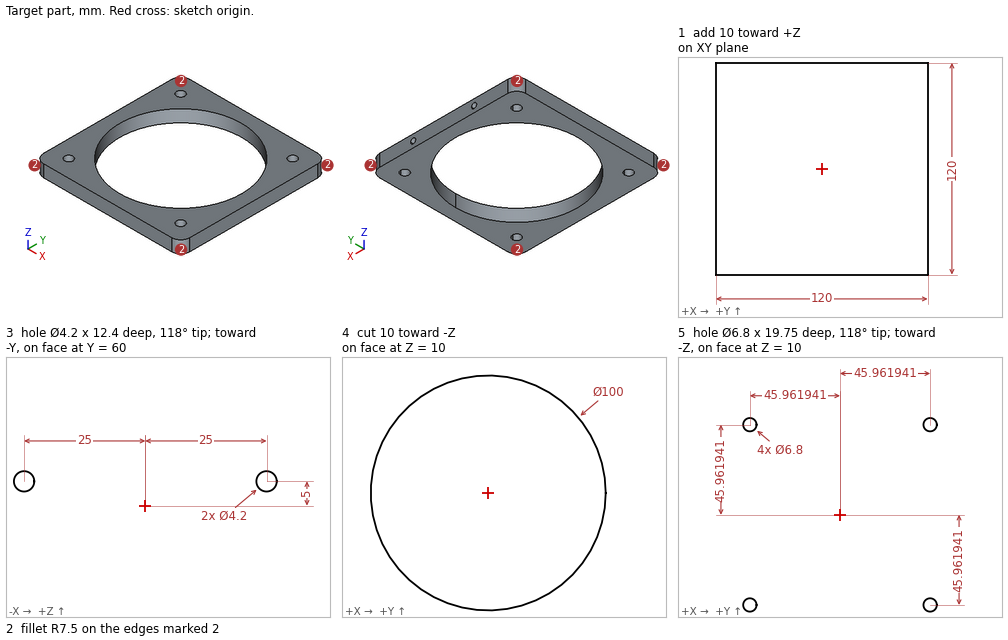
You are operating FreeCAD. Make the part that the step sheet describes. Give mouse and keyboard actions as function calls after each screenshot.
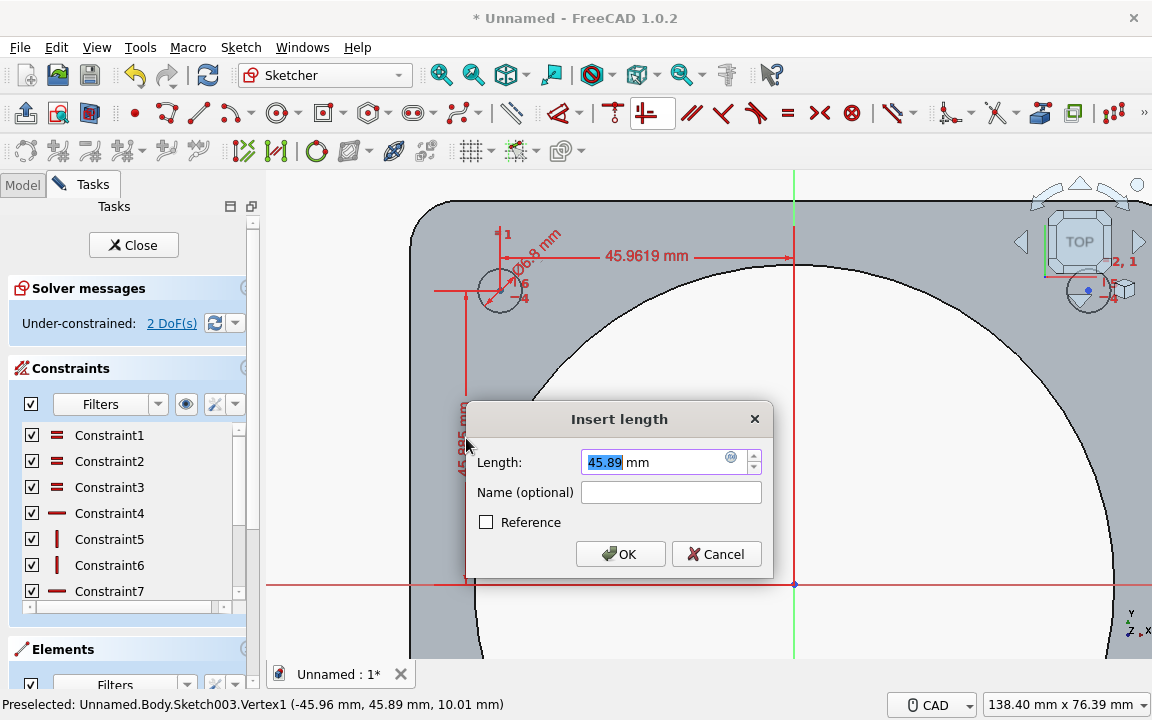
text(45.961941)
key(Return)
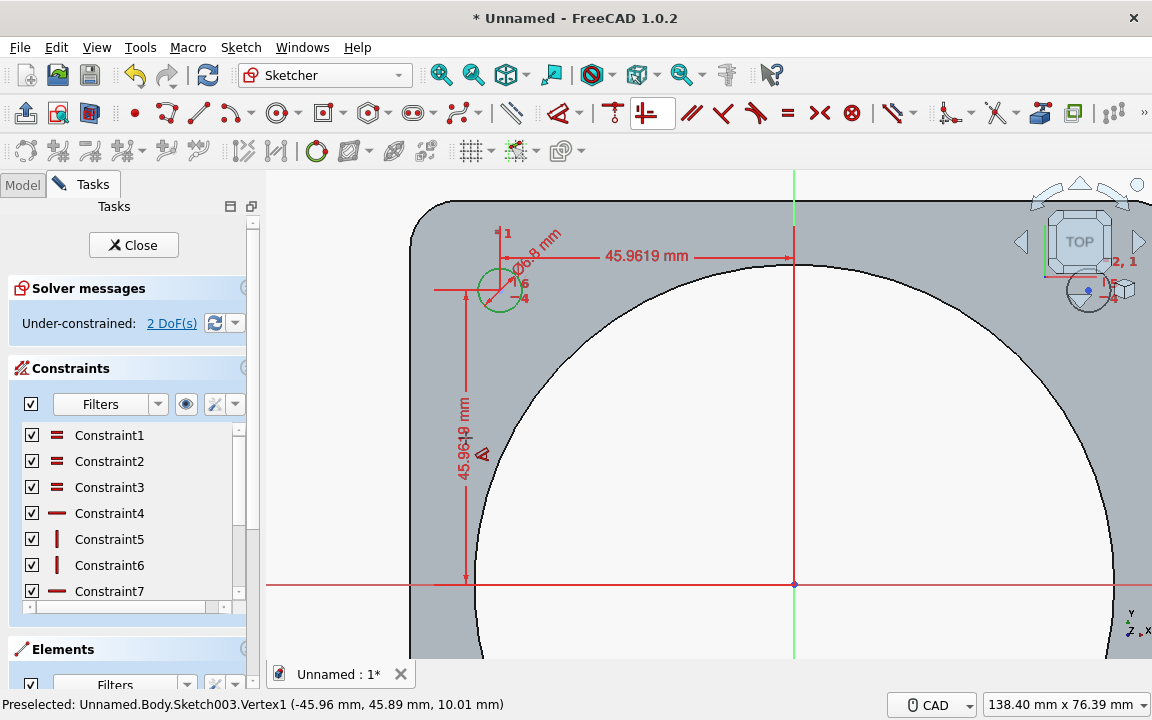
scroll(515, 276, down, 4)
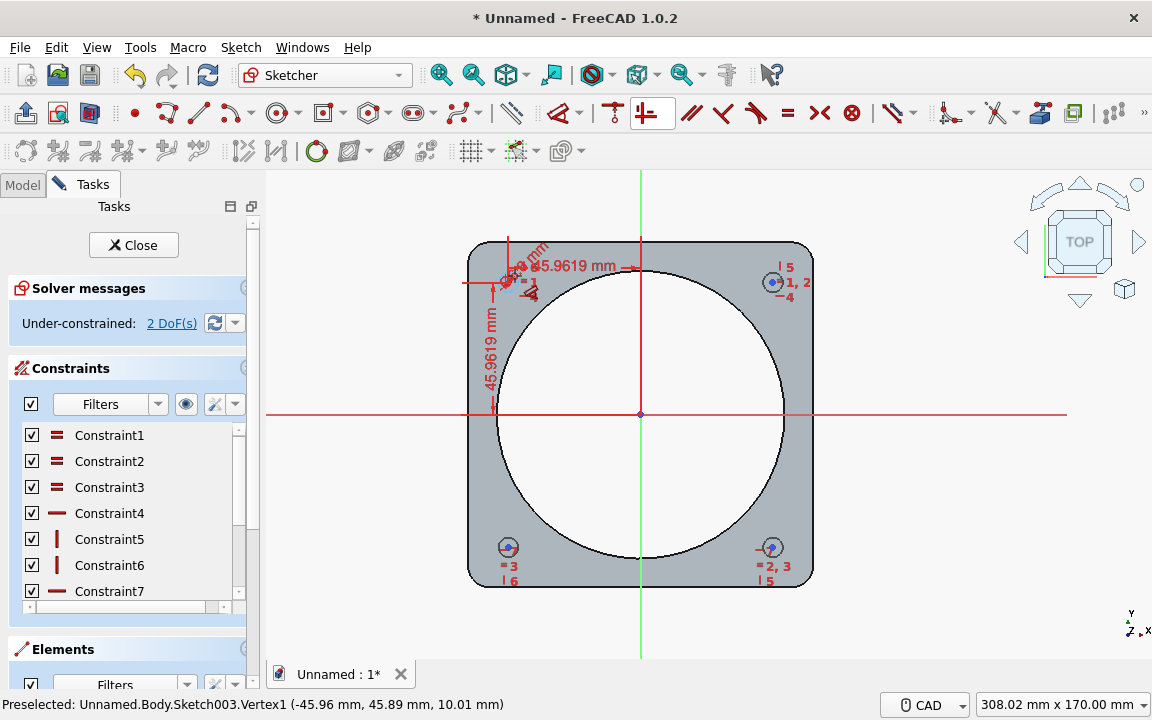
click(773, 283)
click(707, 249)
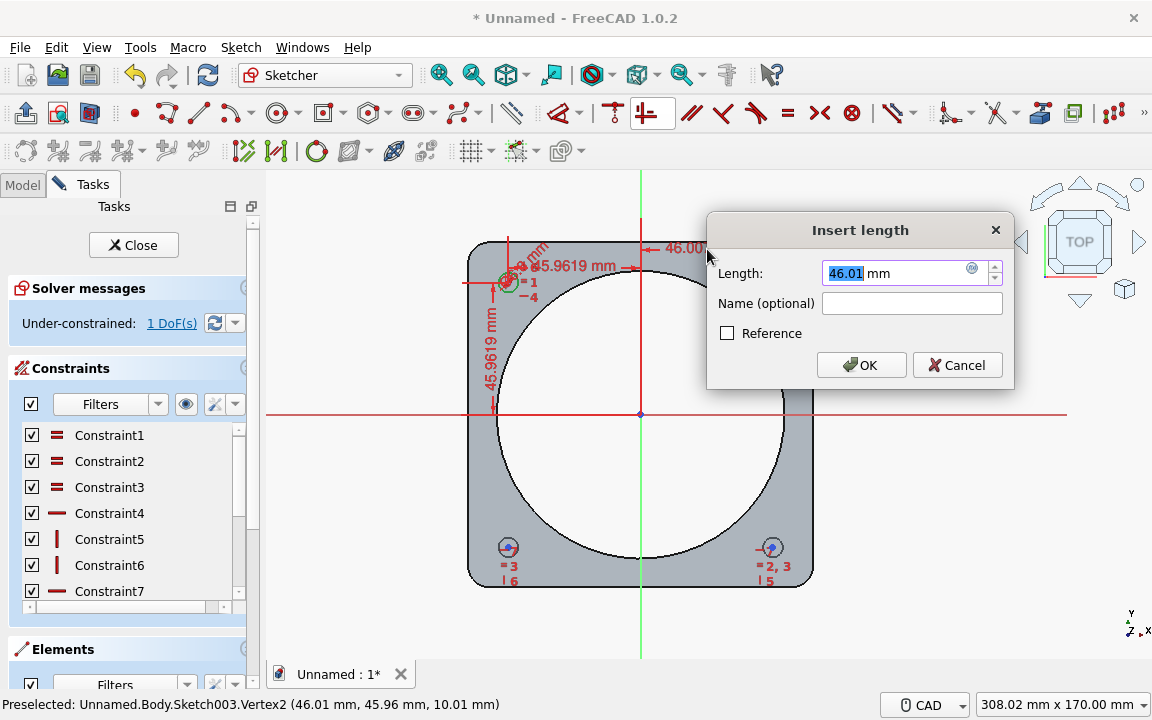
text(45.961941)
key(Return)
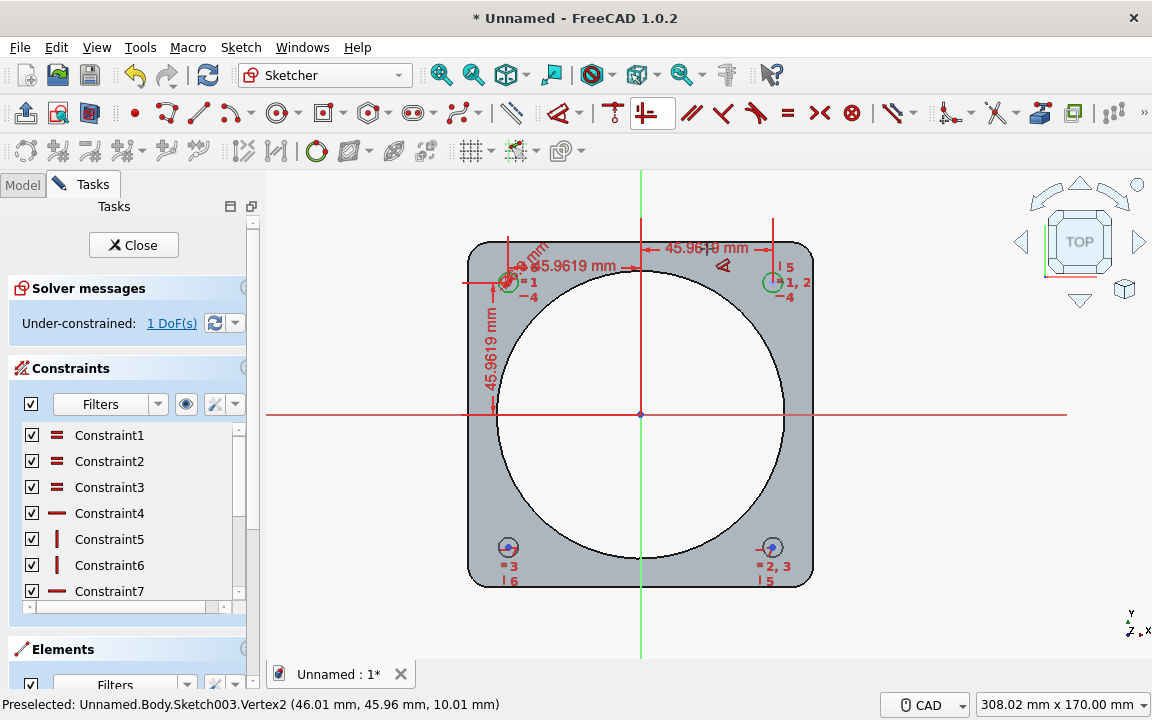
click(773, 547)
click(807, 481)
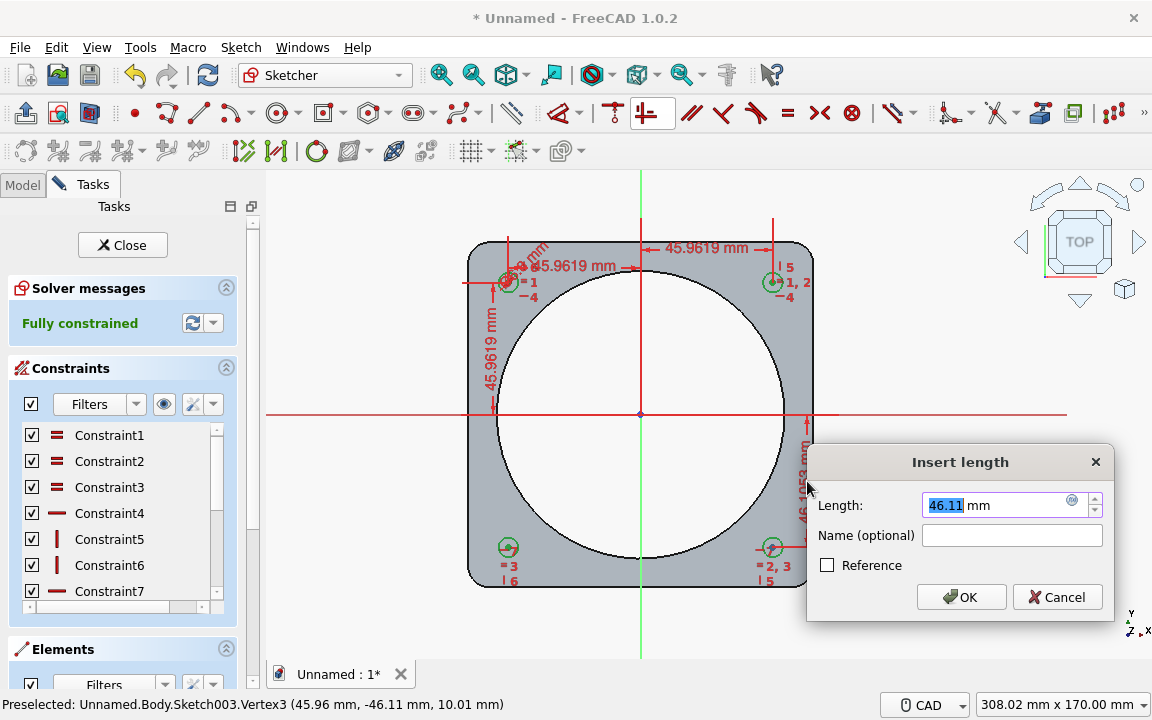
text(45.961941)
key(Return)
key(Escape)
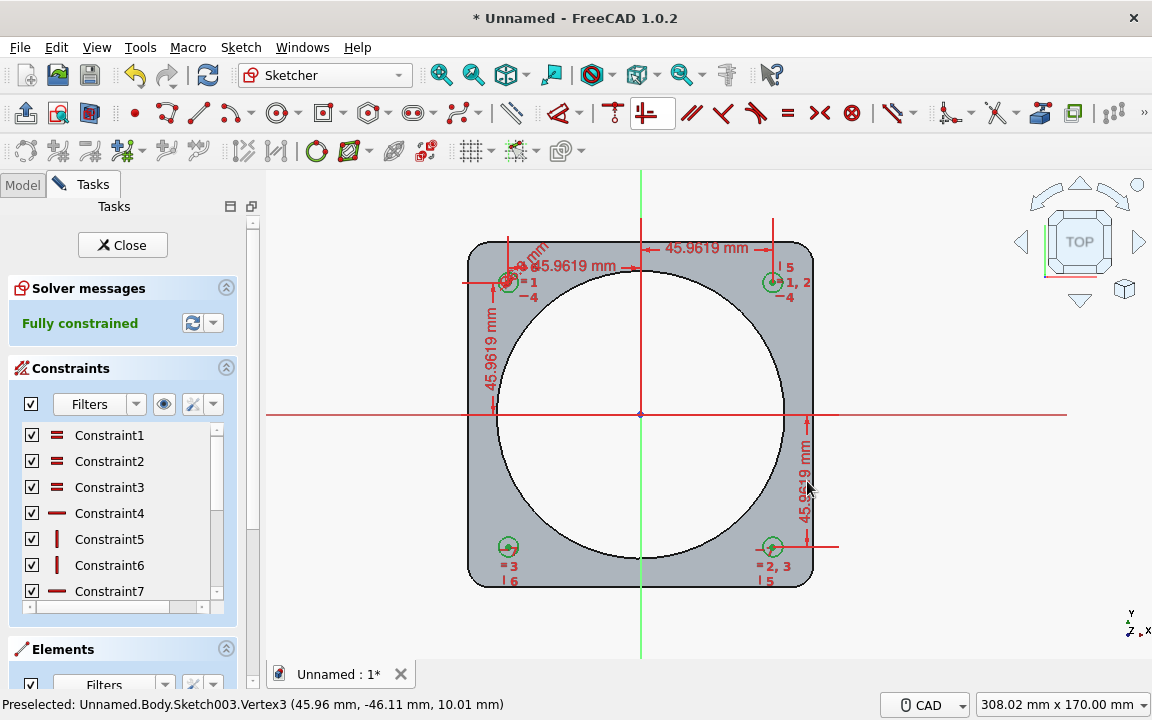
click(123, 245)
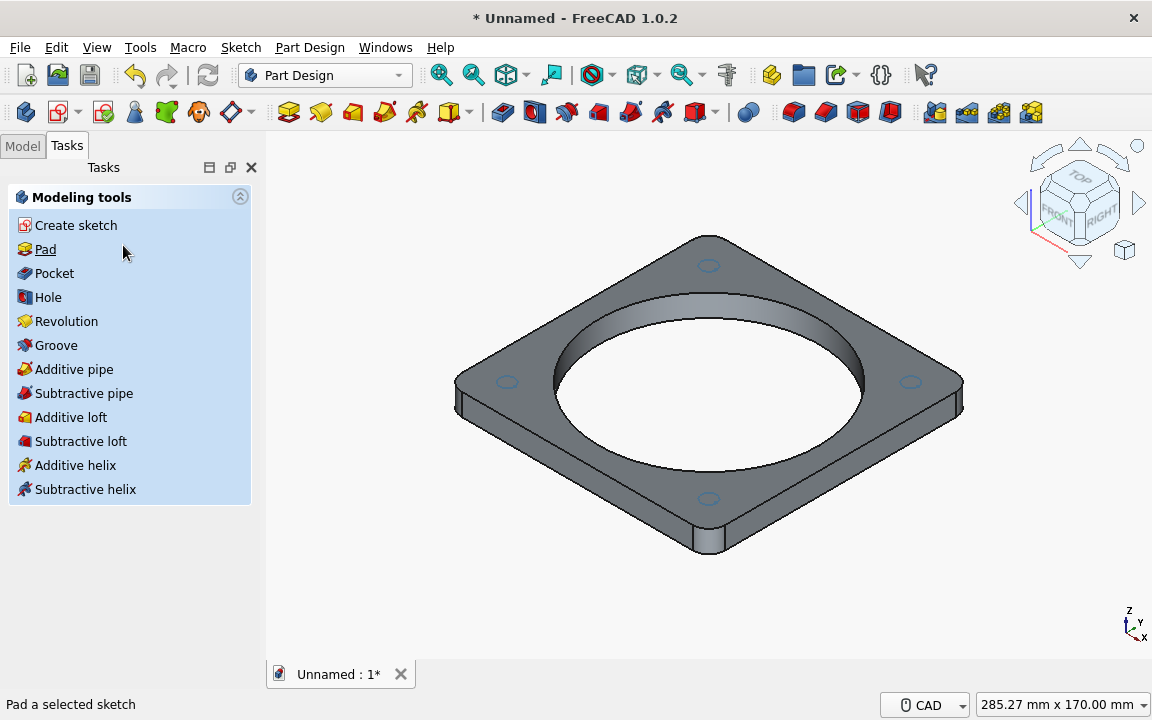
click(536, 112)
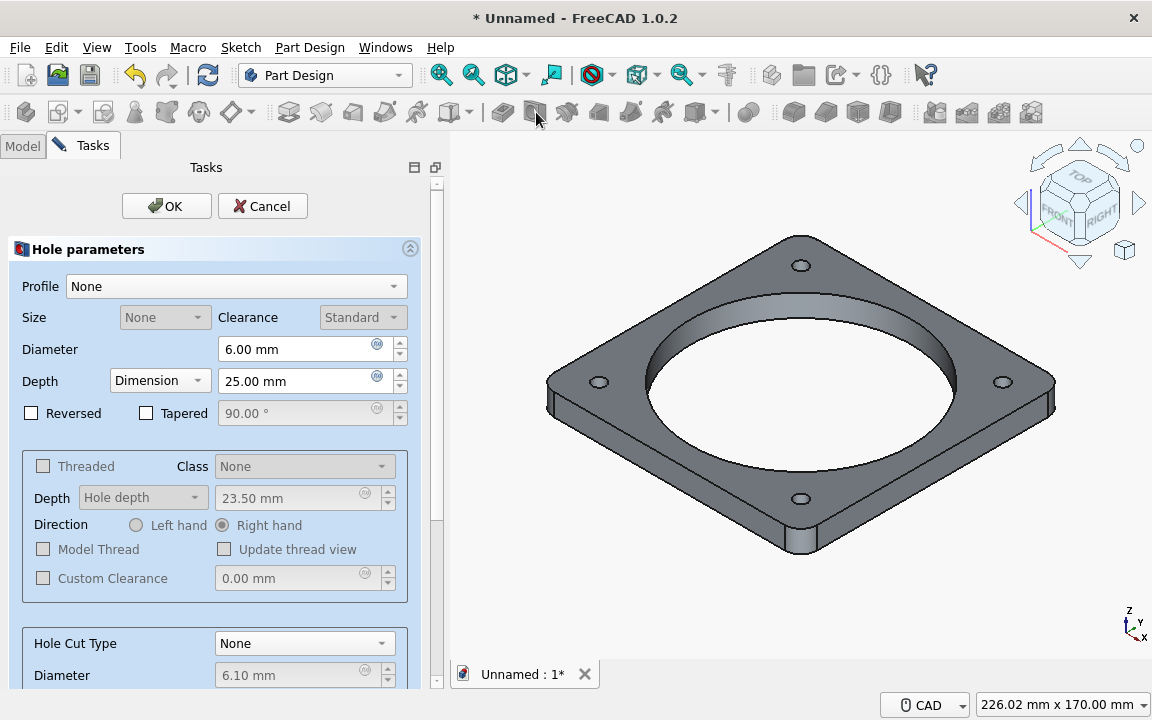
triple_click(305, 349)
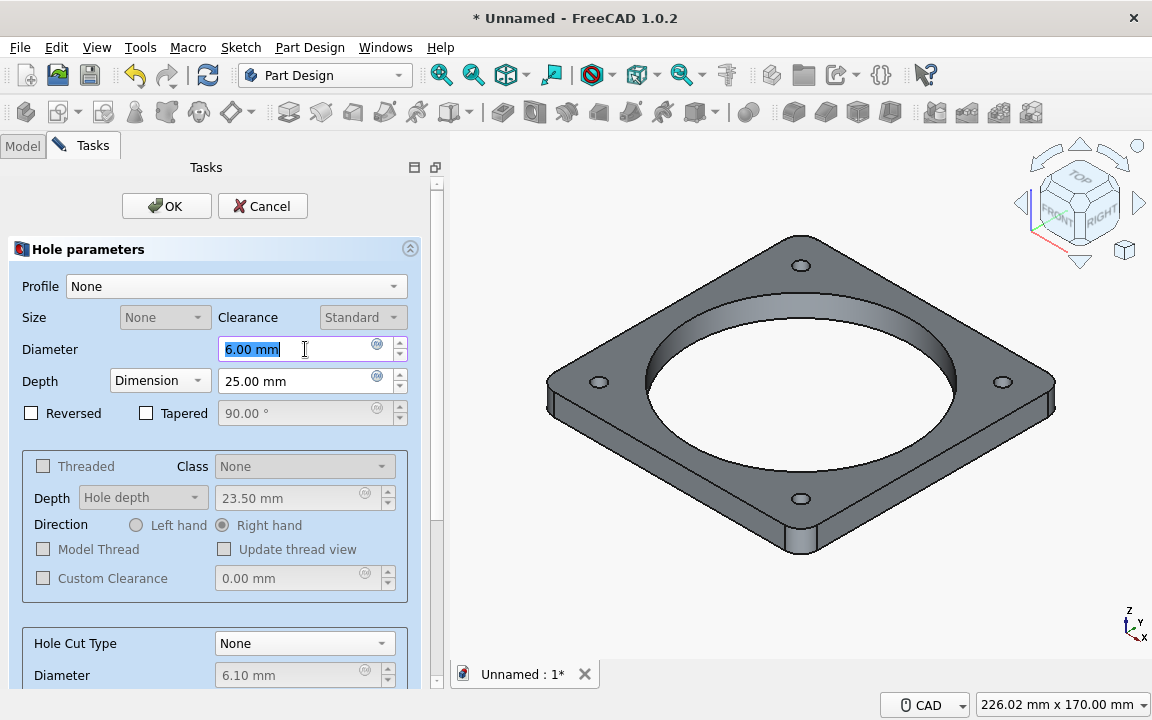
text(6.8)
key(Tab)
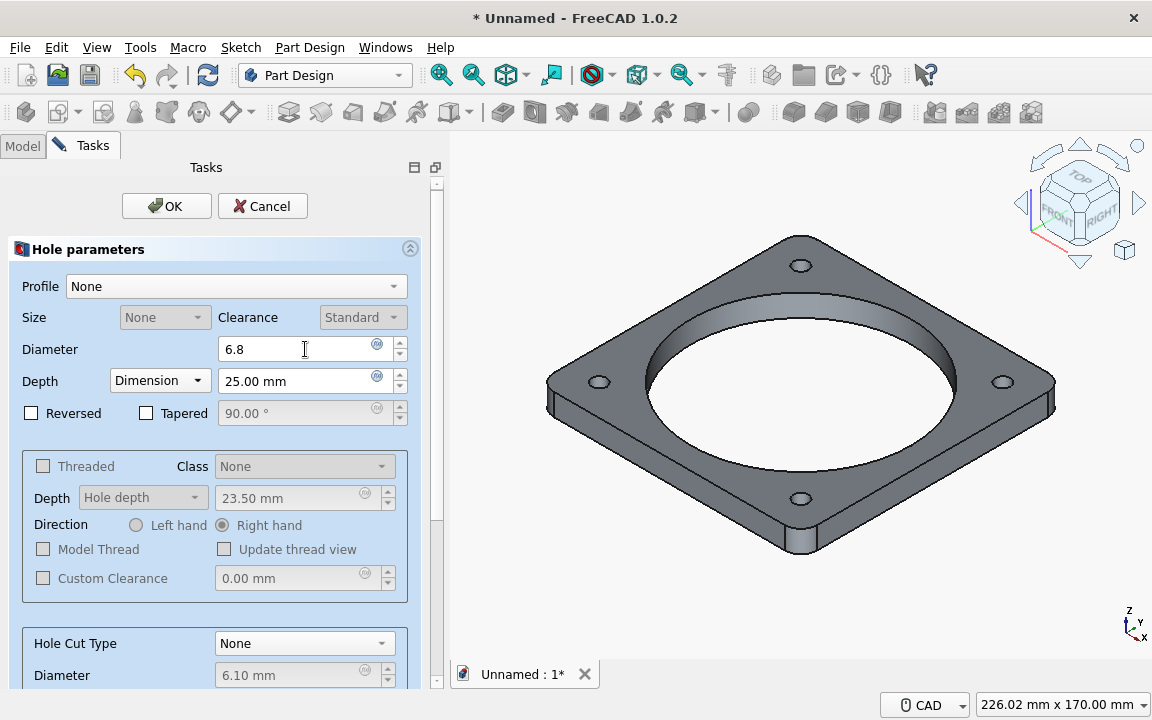
triple_click(305, 381)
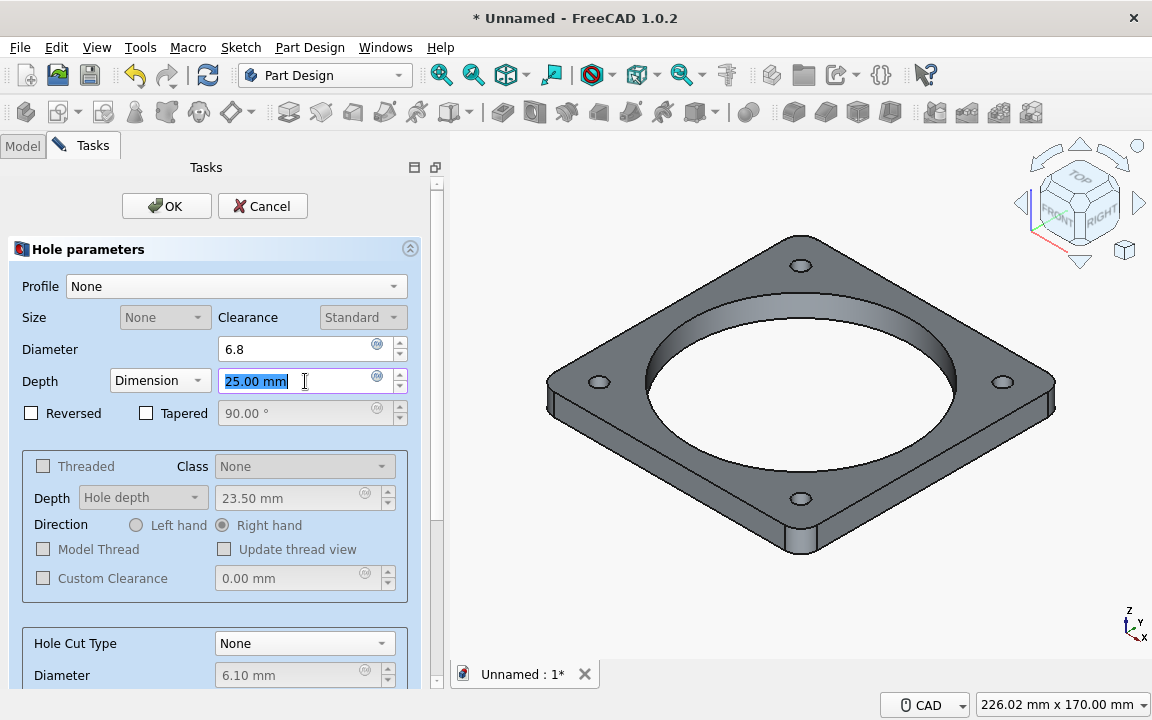
text(19.75)
key(Tab)